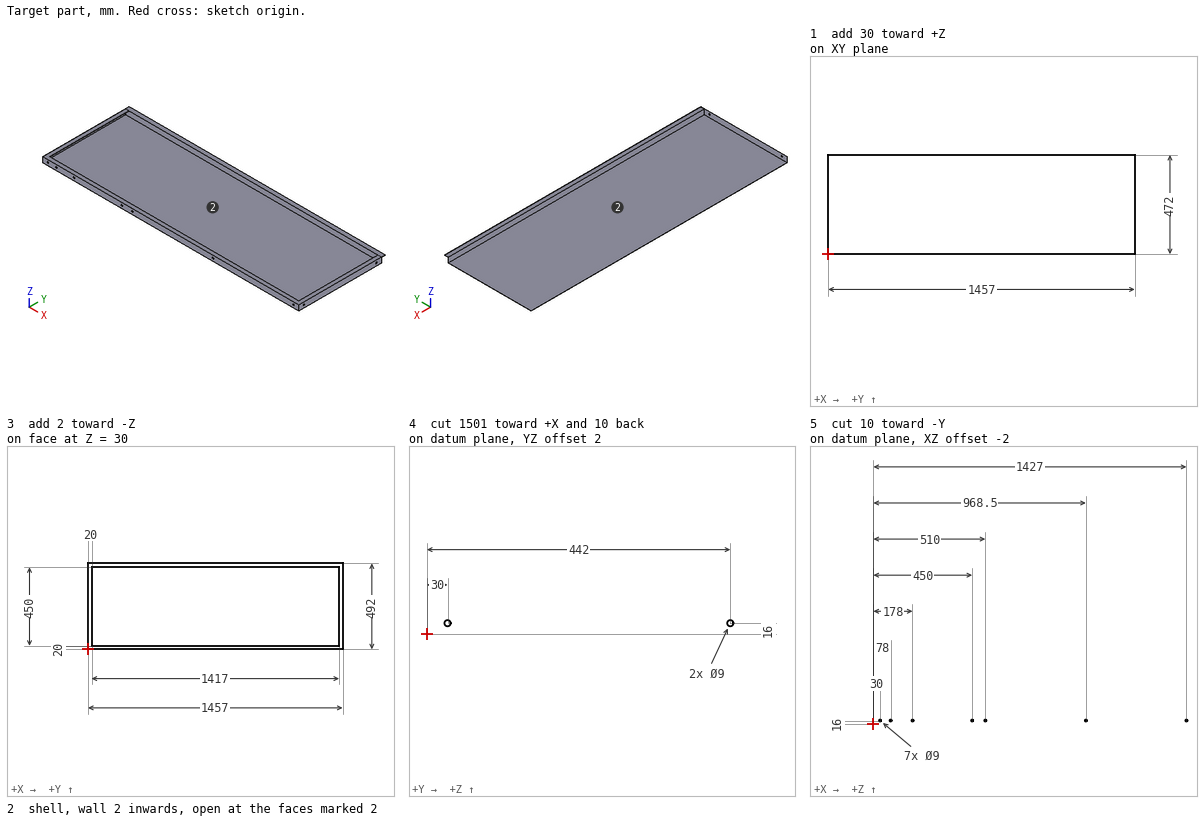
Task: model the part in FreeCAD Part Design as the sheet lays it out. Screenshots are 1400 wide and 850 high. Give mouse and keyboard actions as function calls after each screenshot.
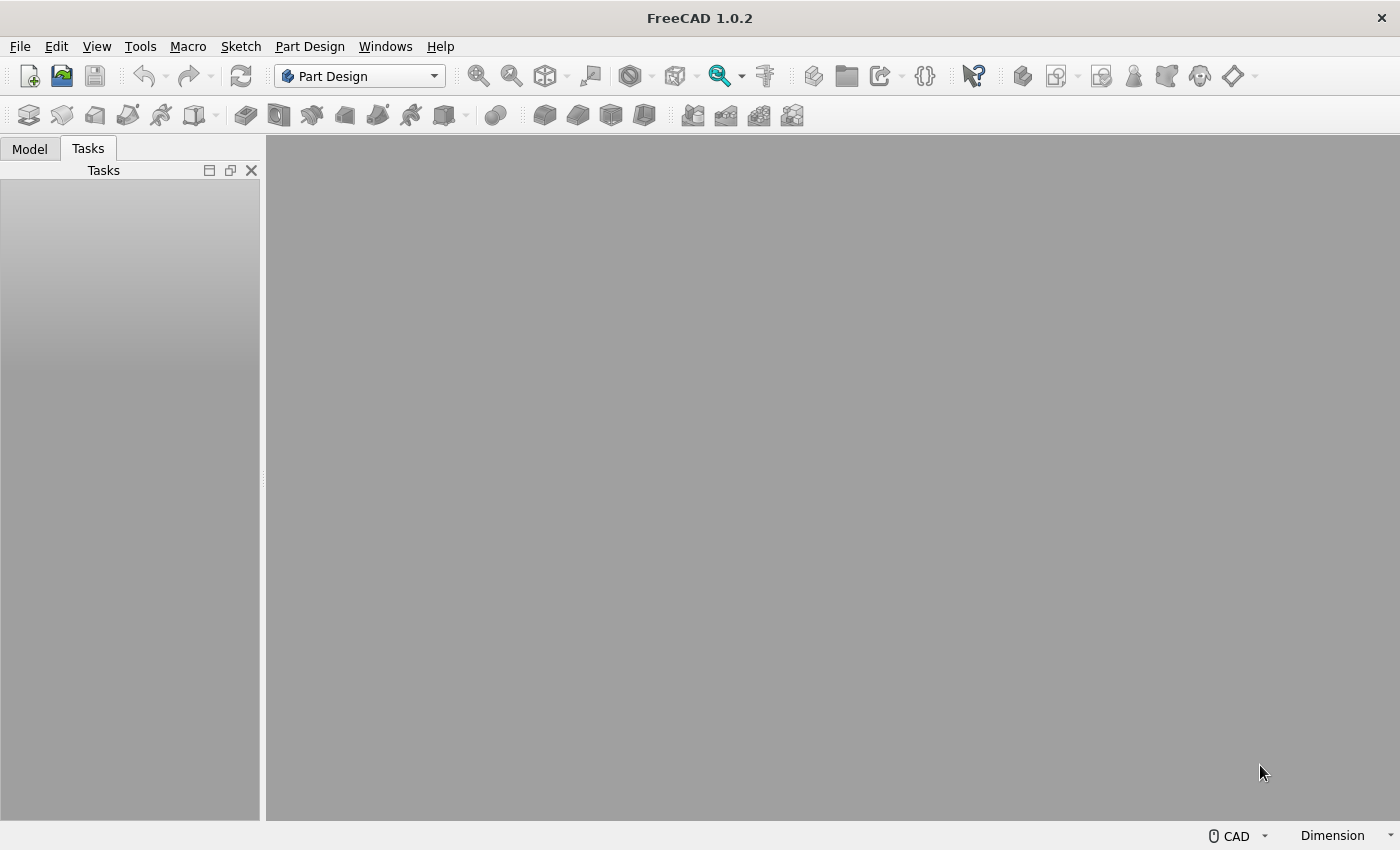
click(29, 76)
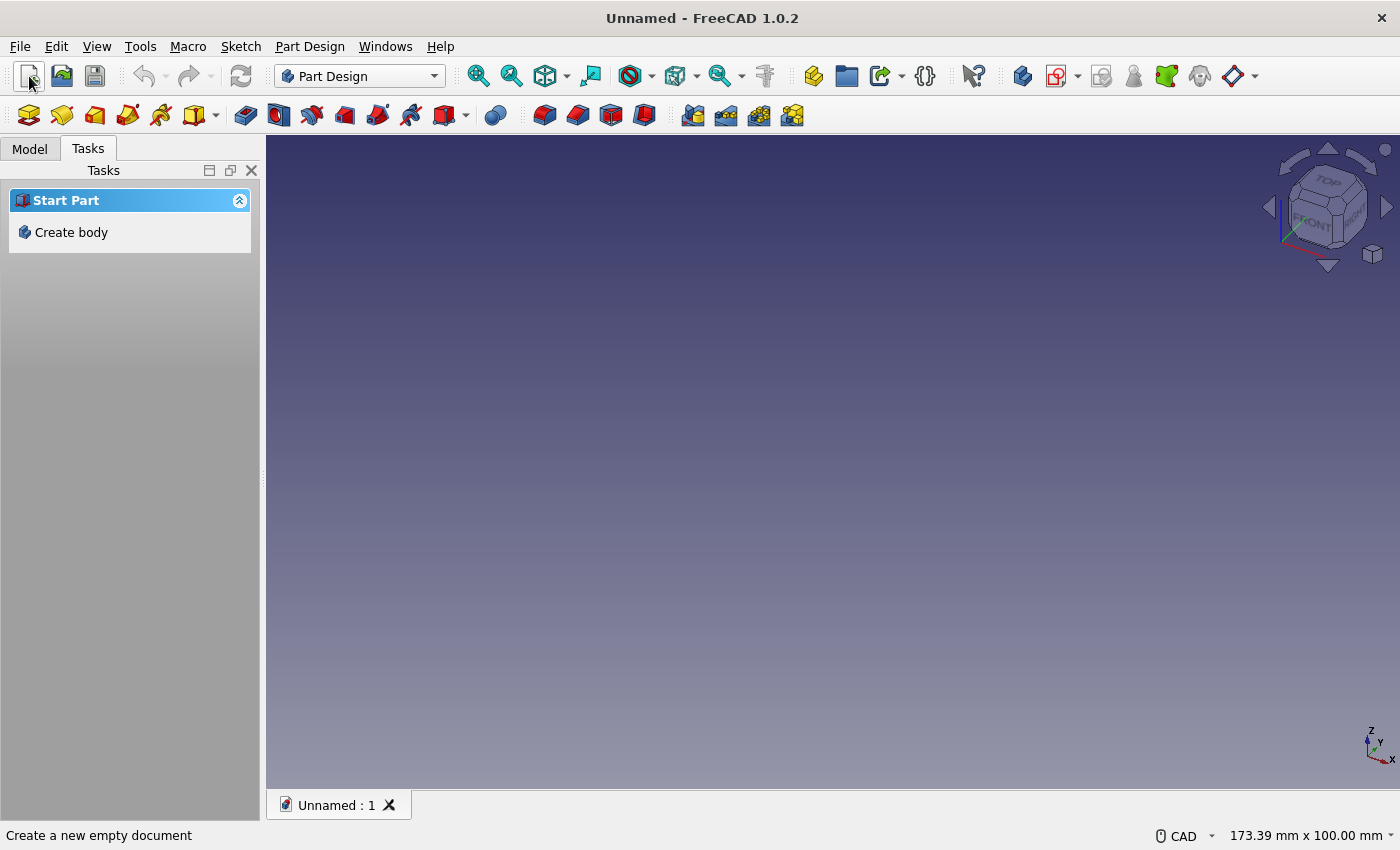
click(1056, 76)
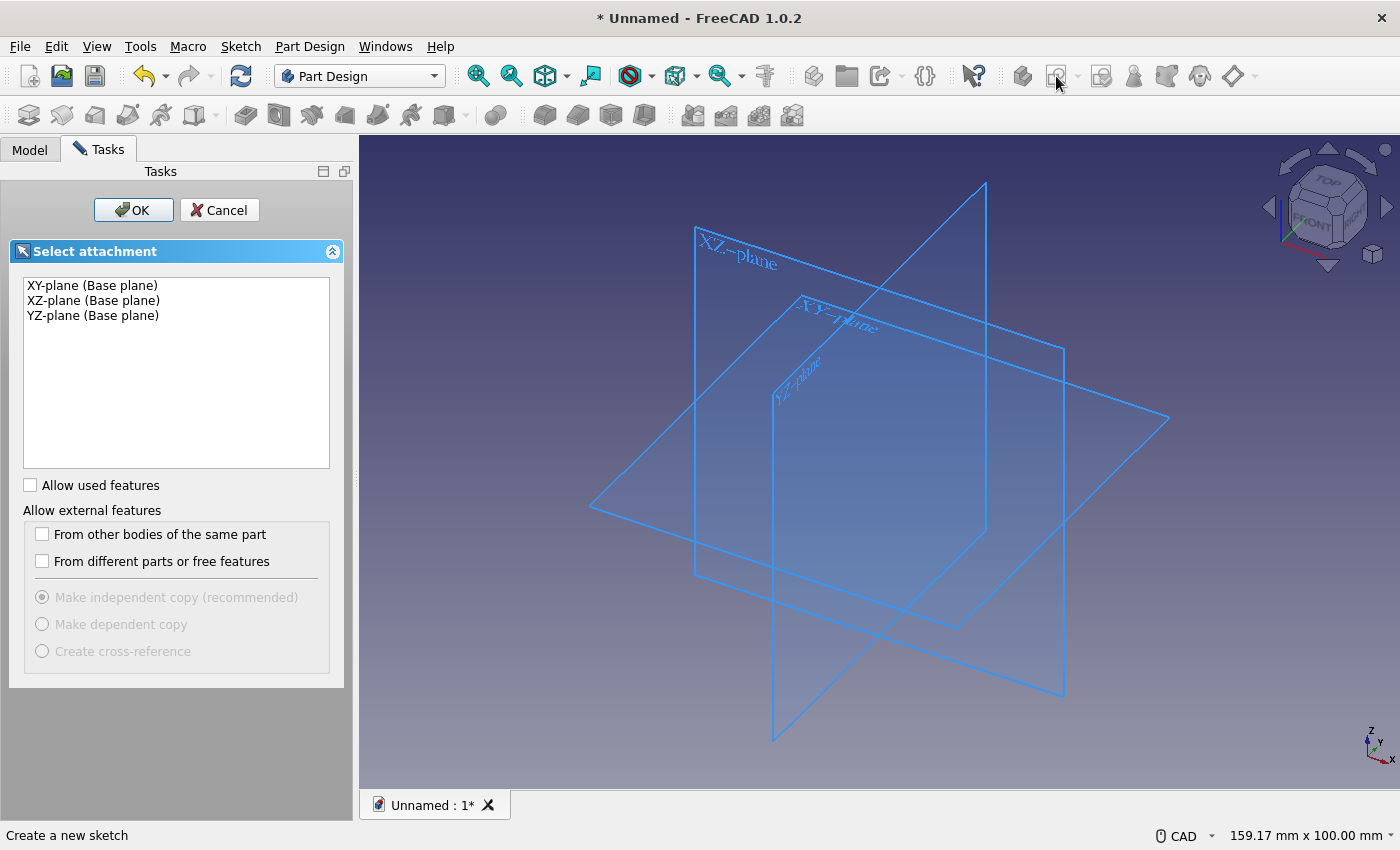
click(84, 286)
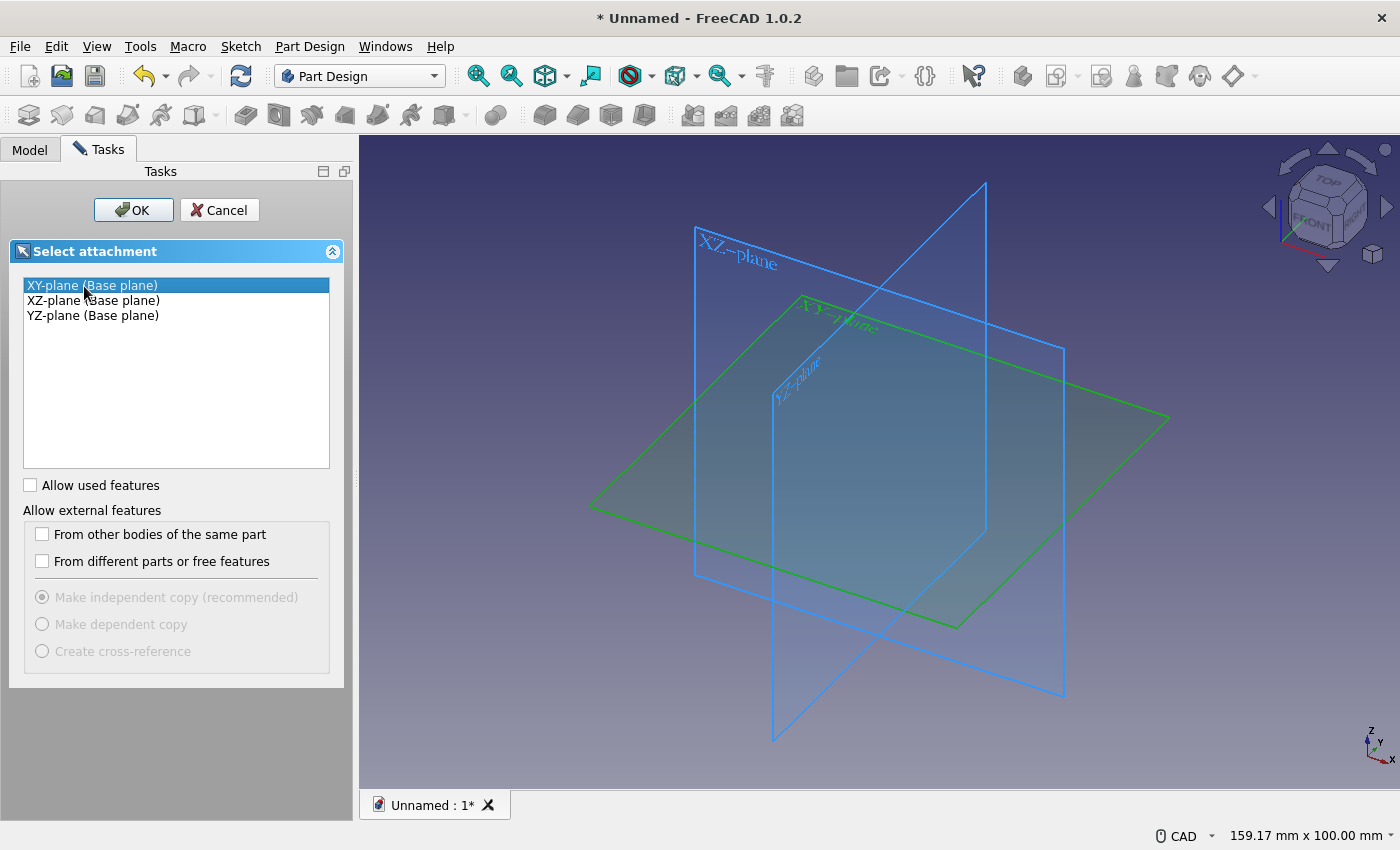
click(134, 210)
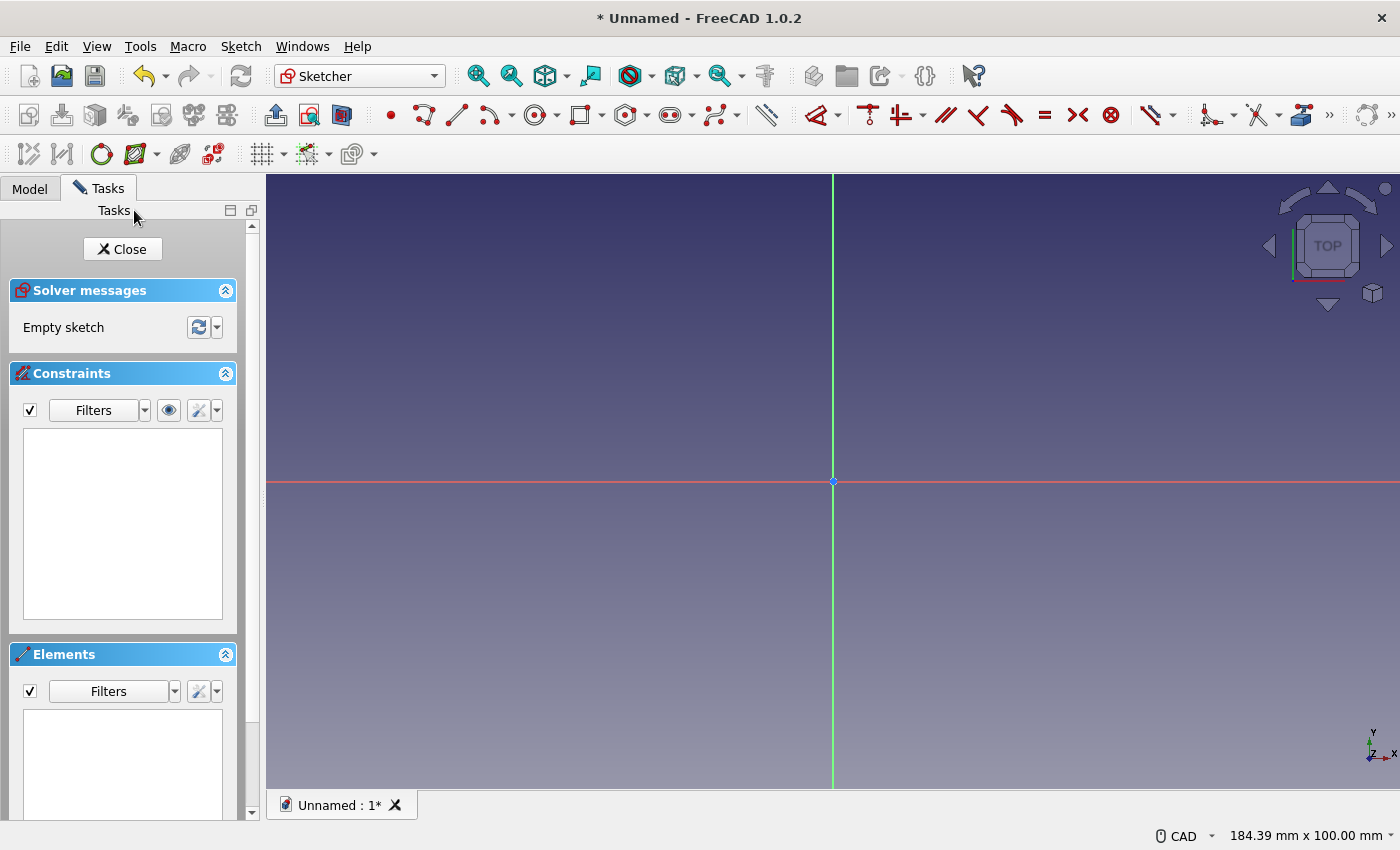
scroll(400, 598, down, 13)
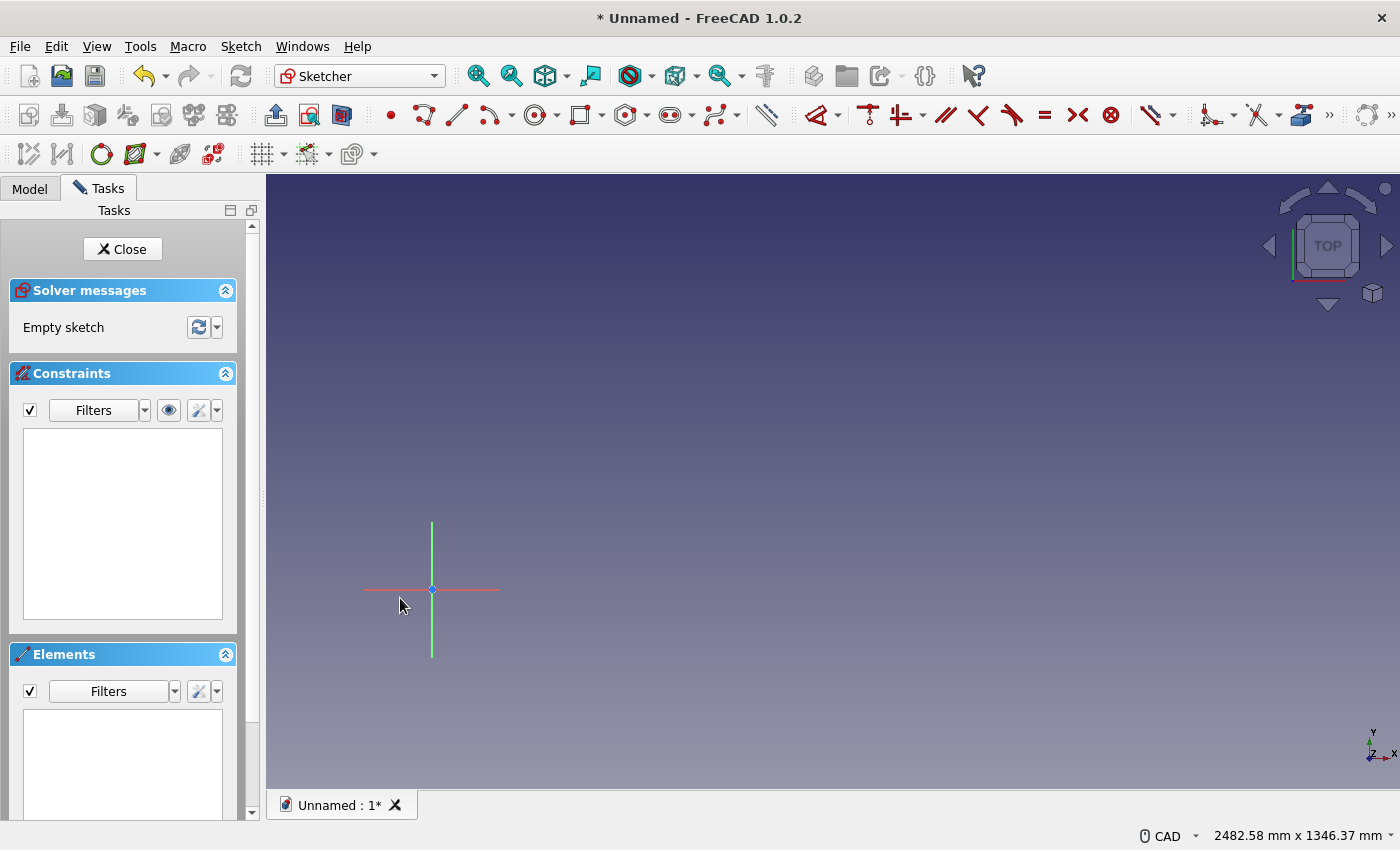
key(g)
key(r)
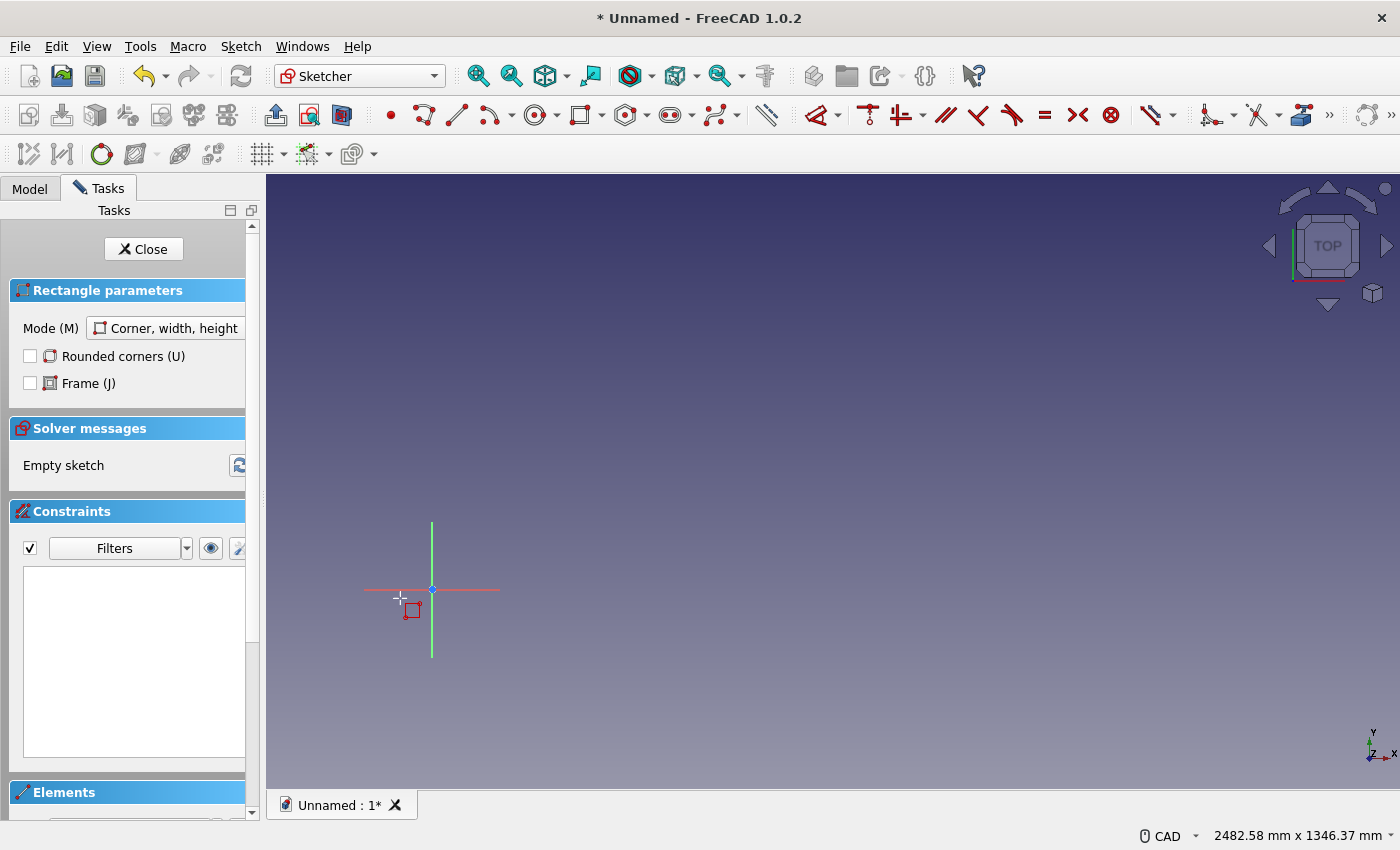
click(432, 590)
move(1098, 374)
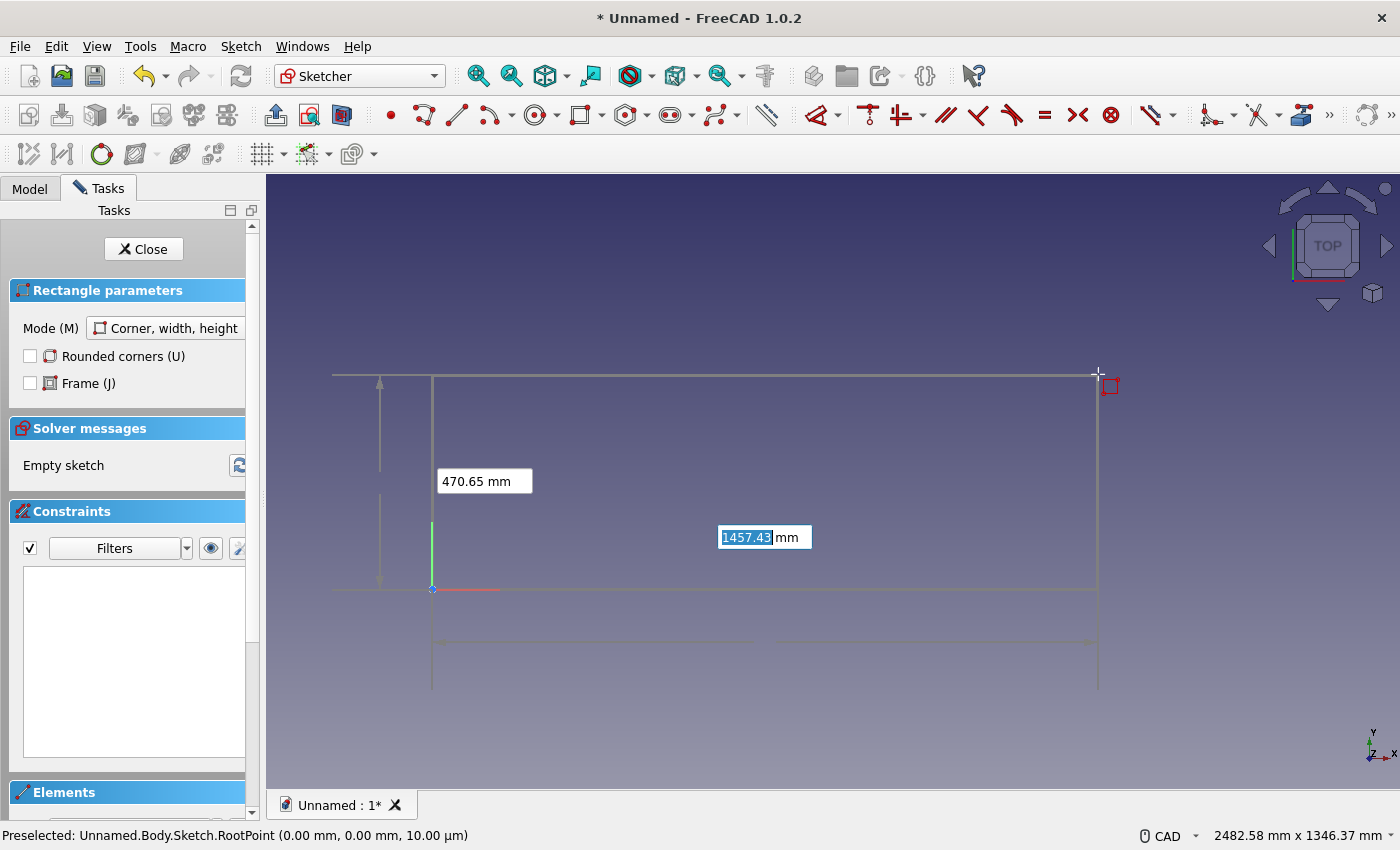
text(1457)
key(Tab)
text(472)
key(Return)
key(Escape)